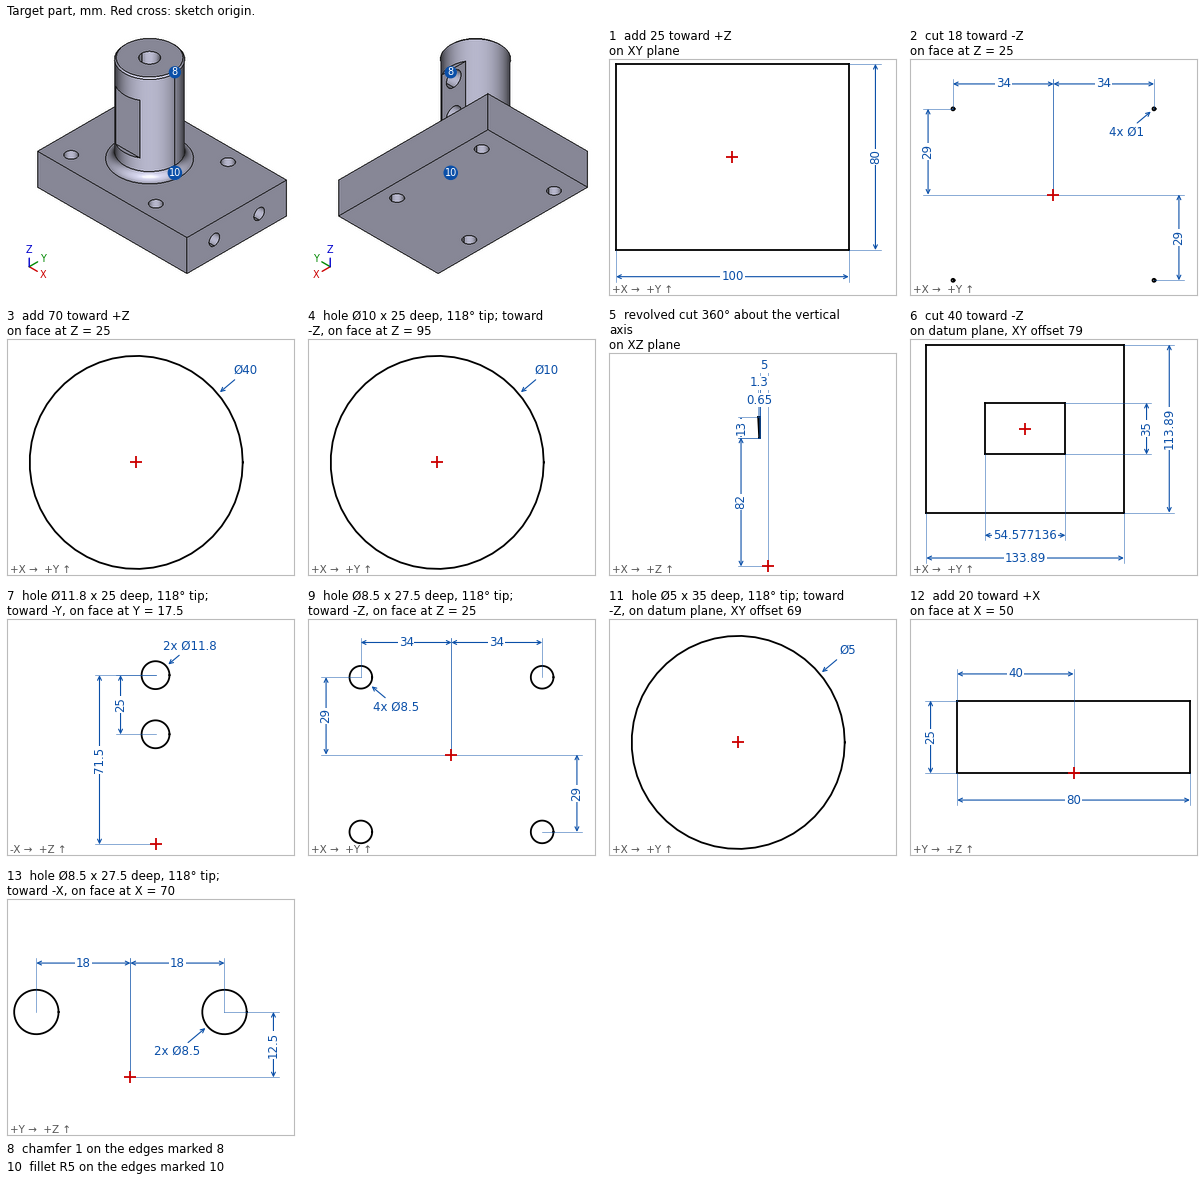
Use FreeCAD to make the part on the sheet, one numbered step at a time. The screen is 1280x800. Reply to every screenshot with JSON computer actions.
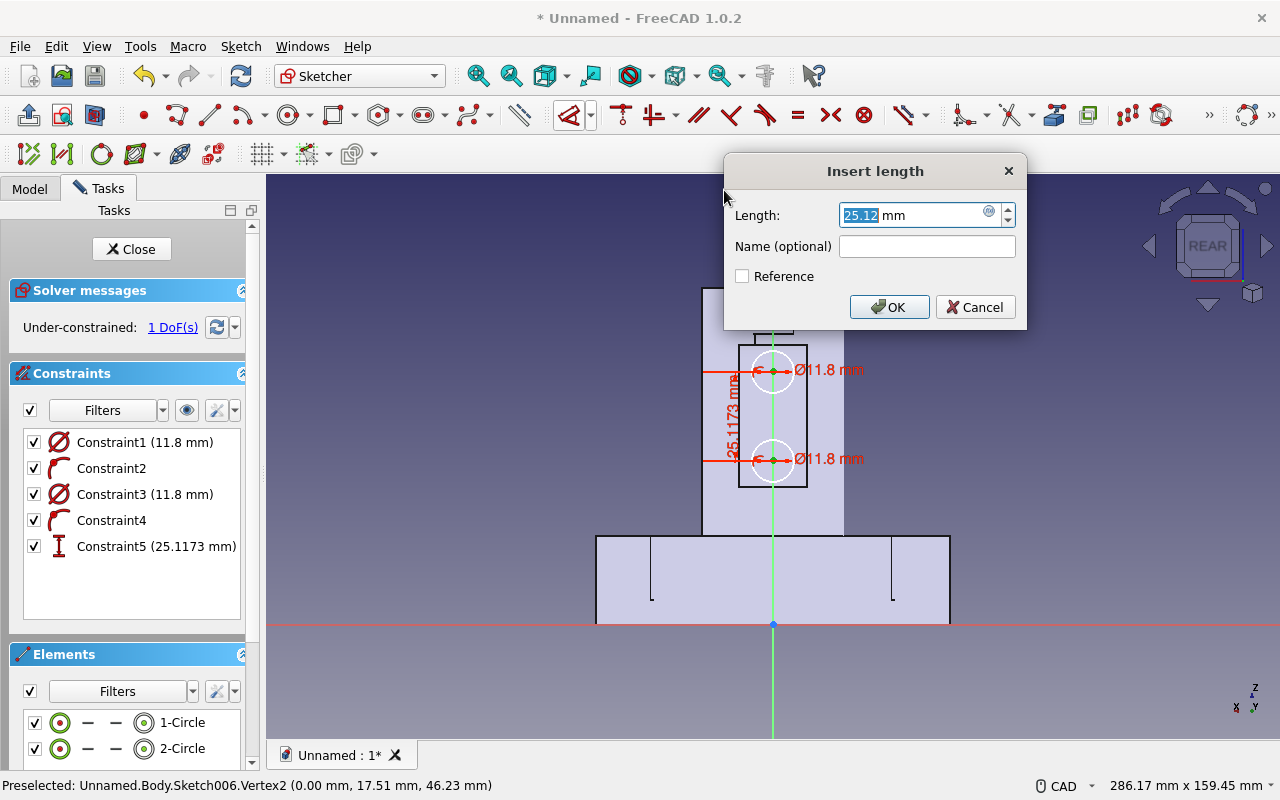
{"action": "type", "text": "25"}
{"action": "key", "text": "Return"}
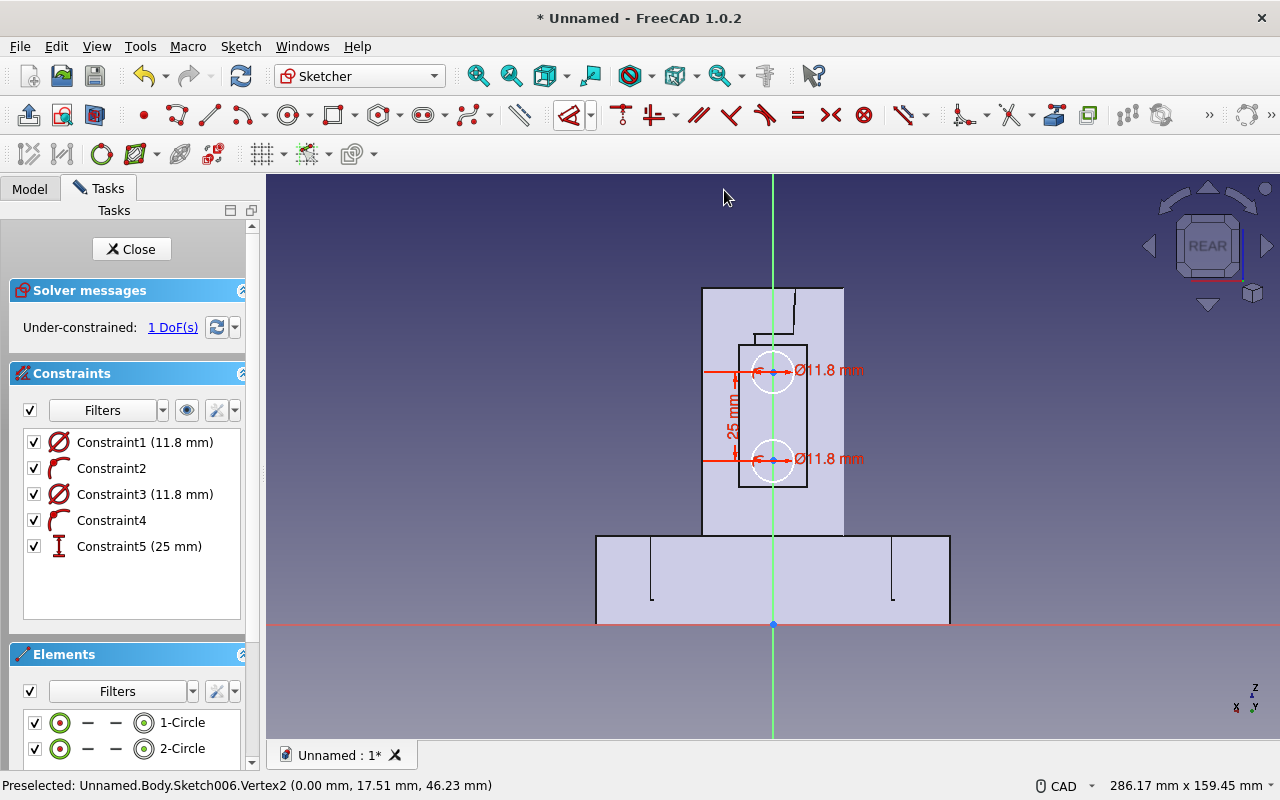
{"action": "left_click", "coordinate": [773, 372]}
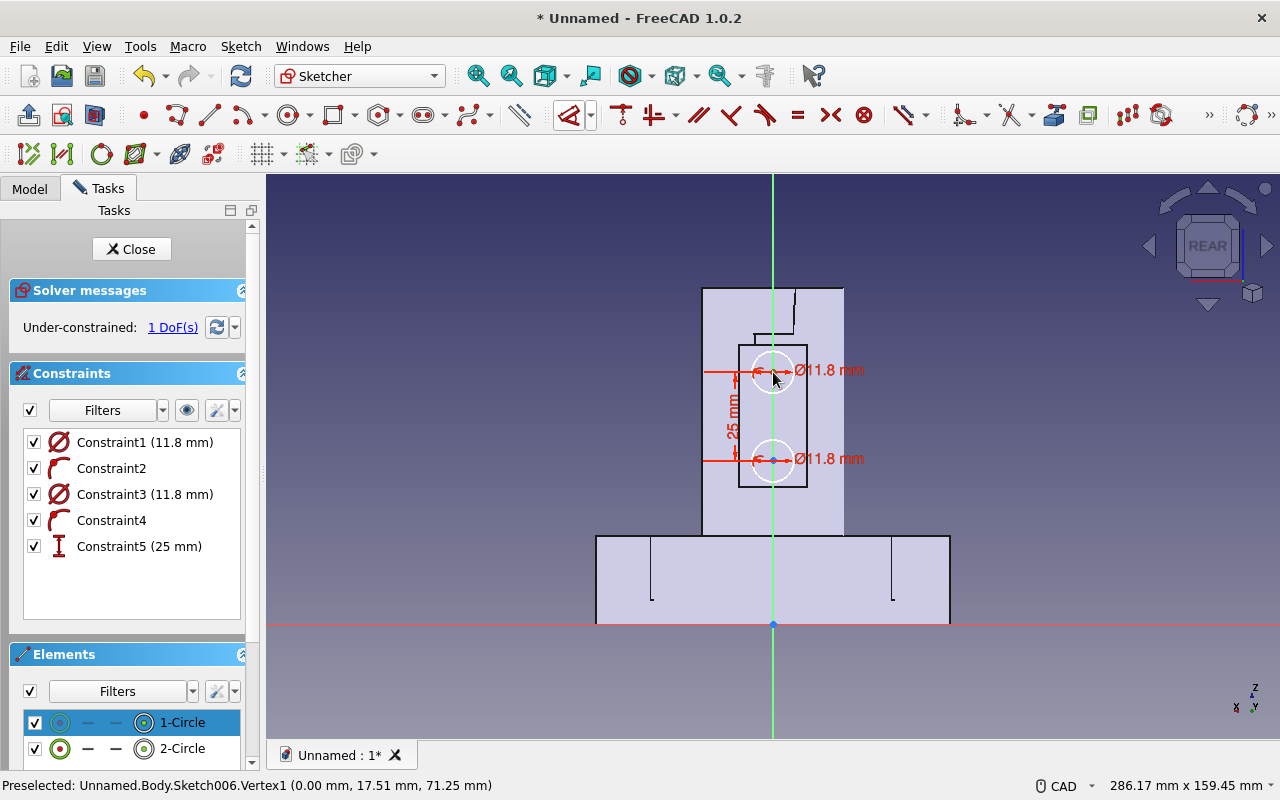
{"action": "left_click", "coordinate": [590, 116]}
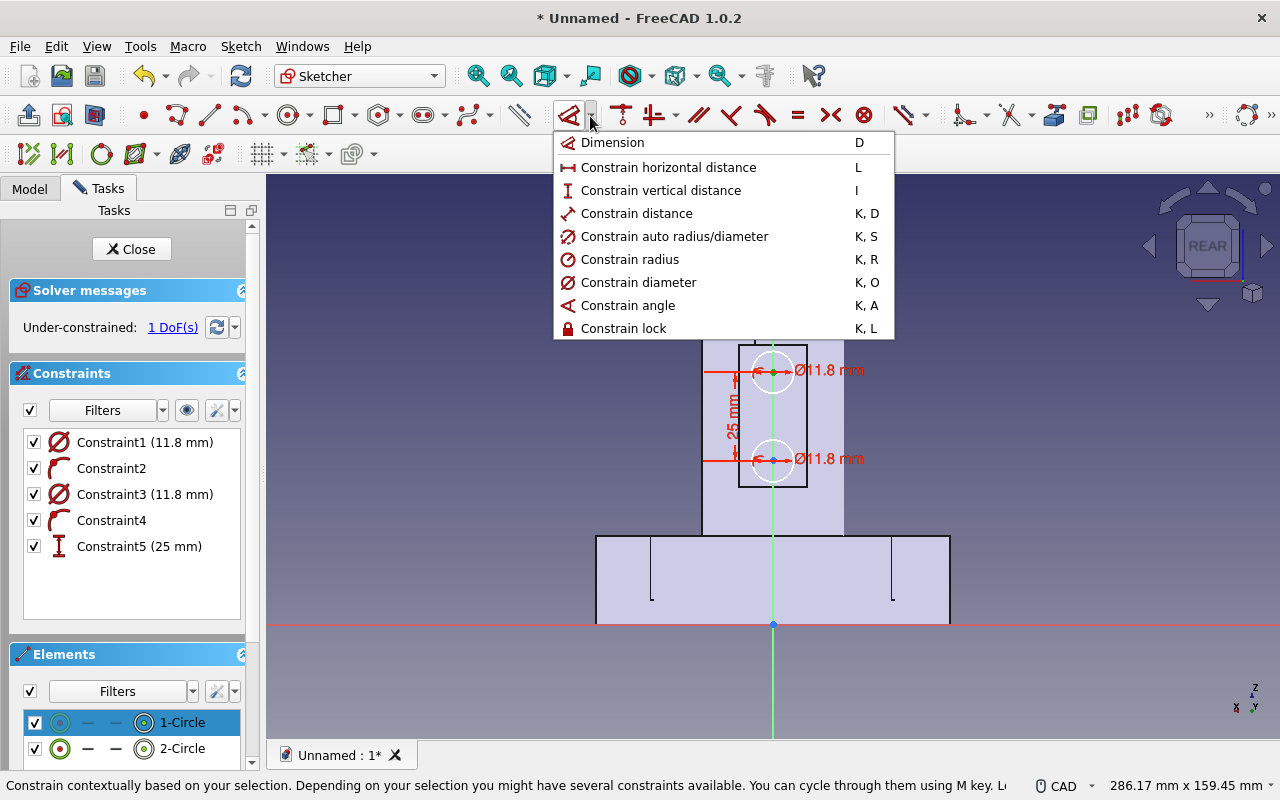
{"action": "left_click", "coordinate": [724, 190]}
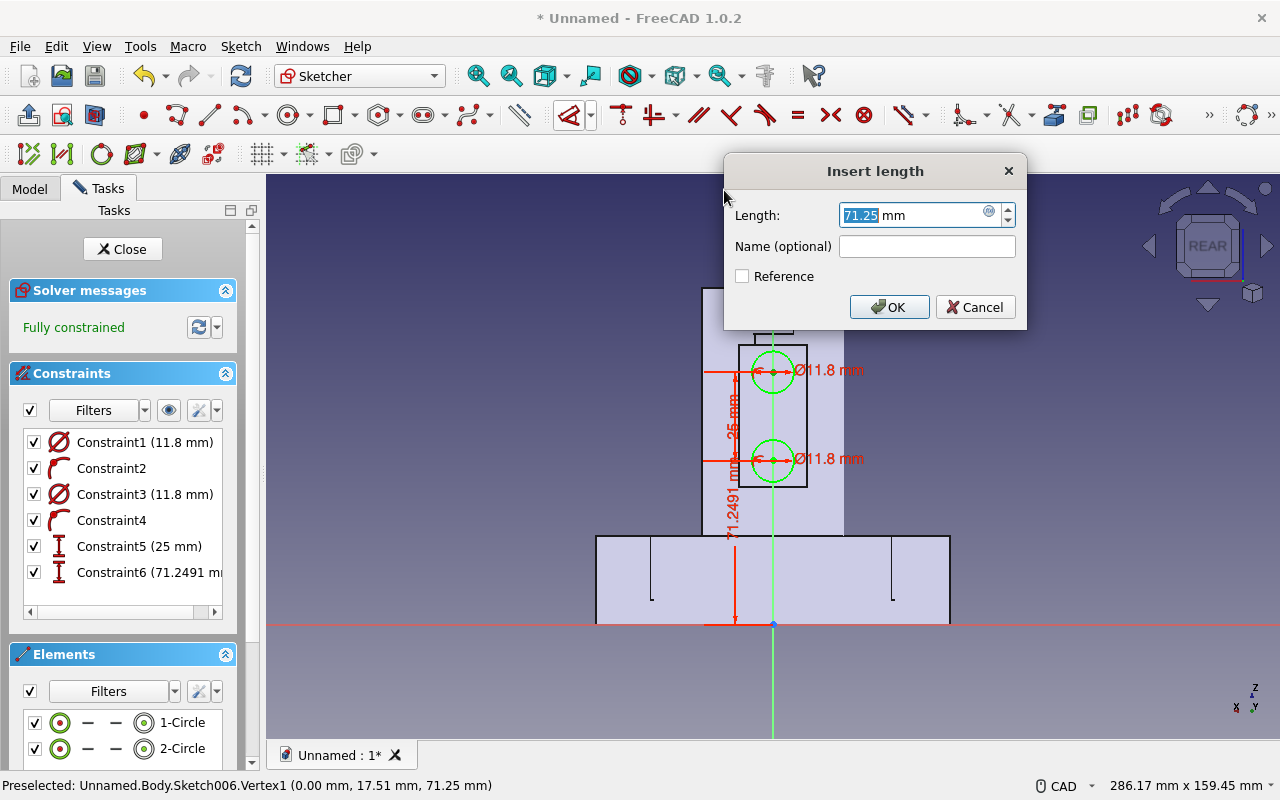
{"action": "type", "text": "71.5"}
{"action": "key", "text": "Return"}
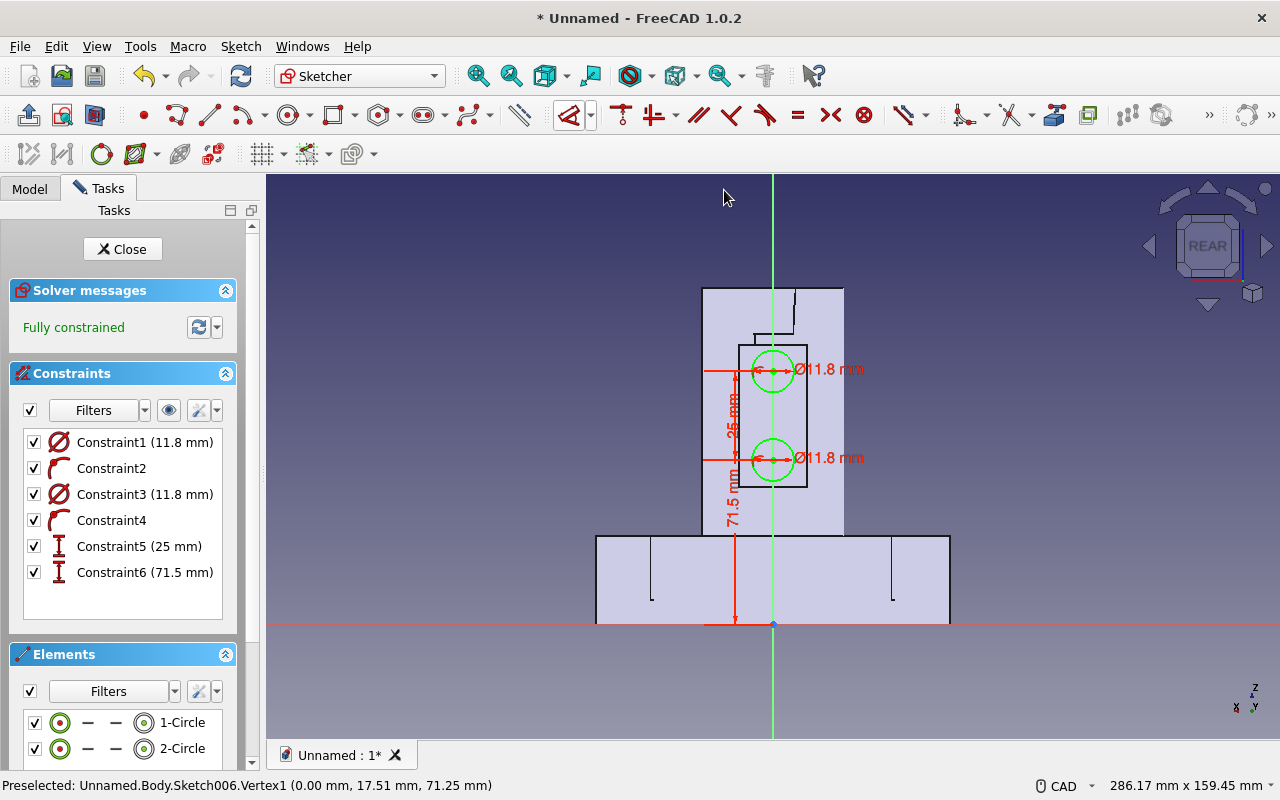
{"action": "left_click", "coordinate": [123, 249]}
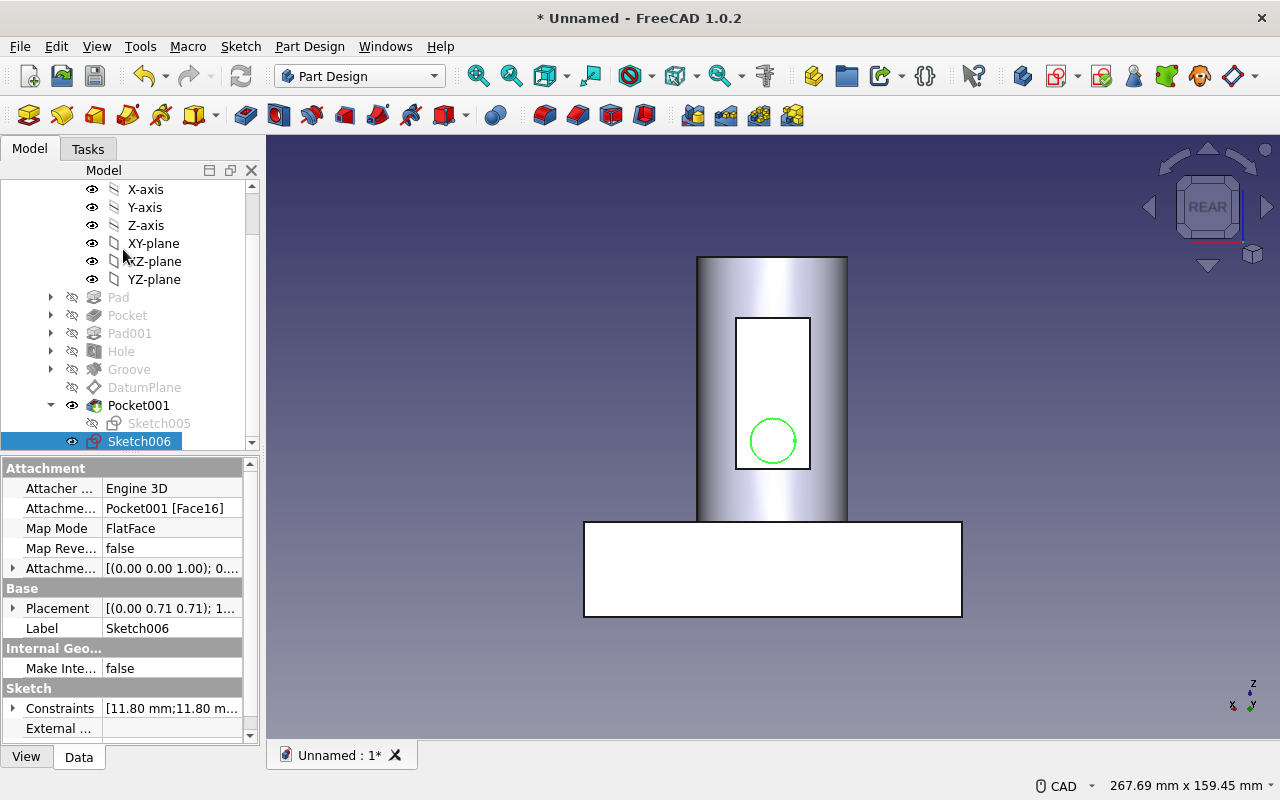
{"action": "left_click", "coordinate": [279, 116]}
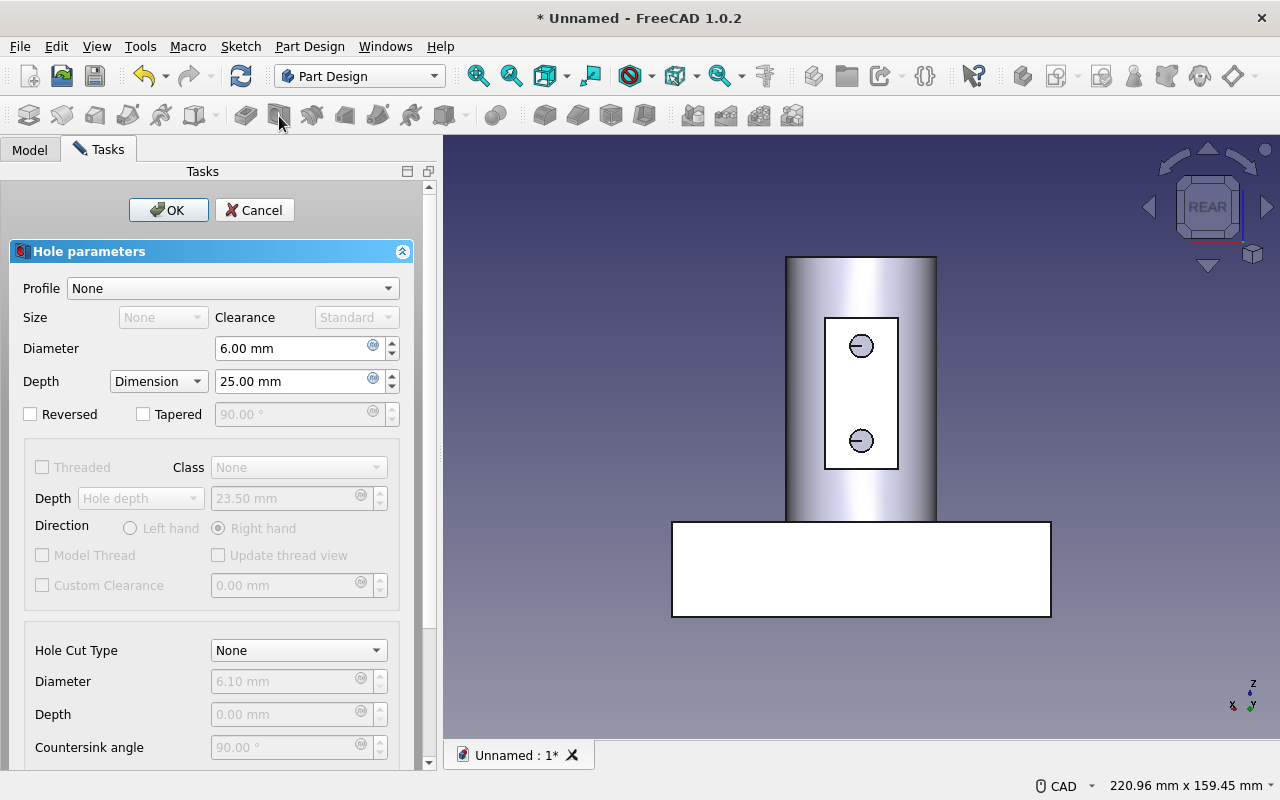
{"action": "triple_click", "coordinate": [300, 348]}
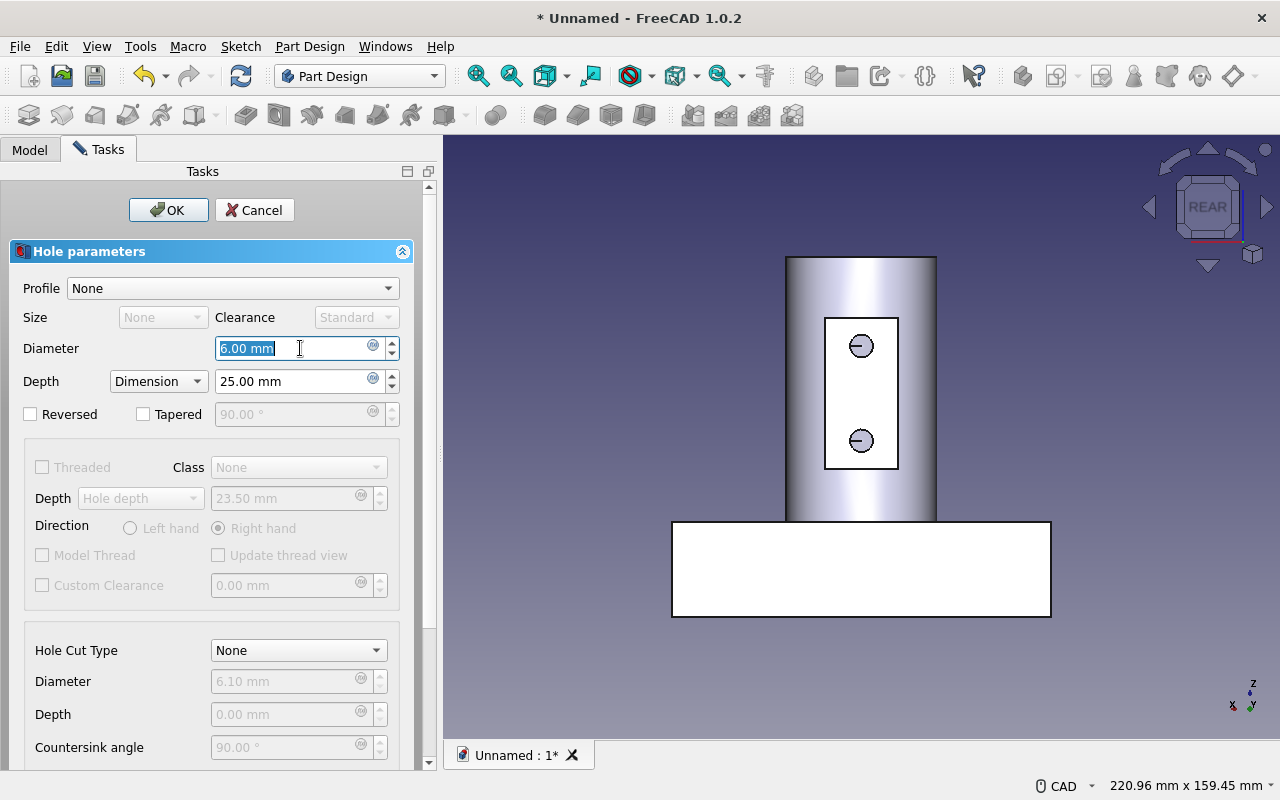
{"action": "type", "text": "11.8"}
{"action": "key", "text": "Tab"}